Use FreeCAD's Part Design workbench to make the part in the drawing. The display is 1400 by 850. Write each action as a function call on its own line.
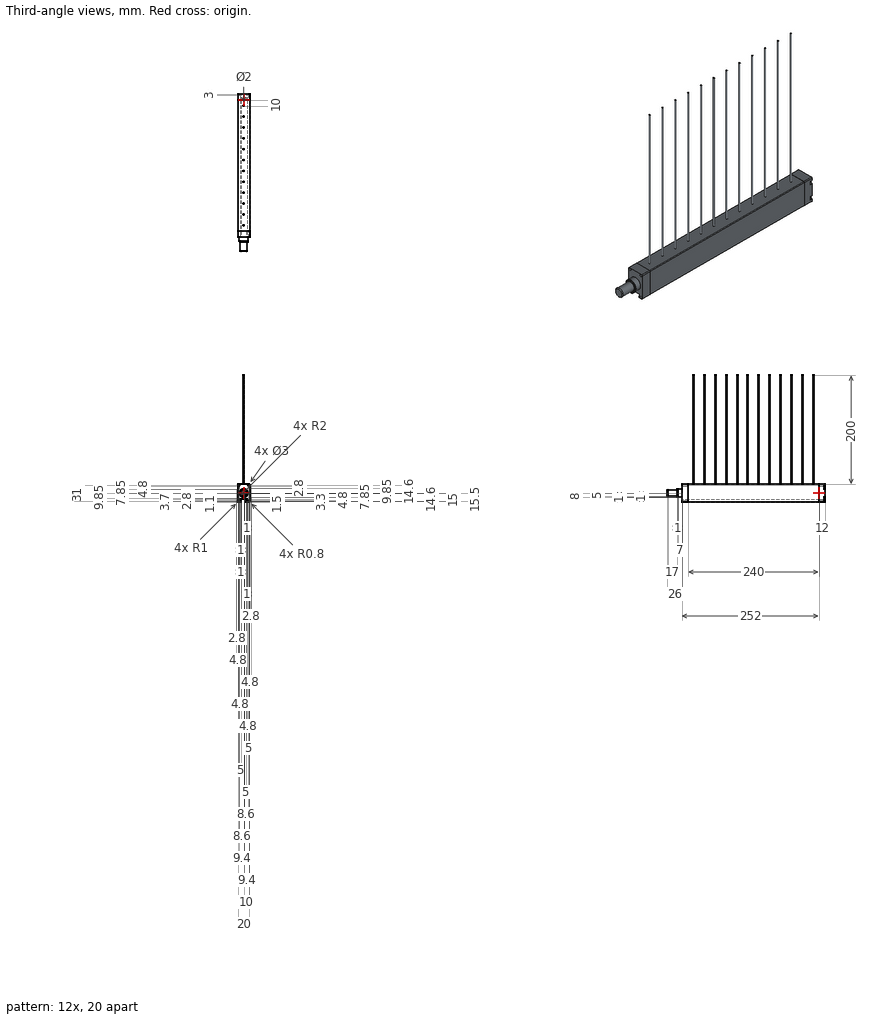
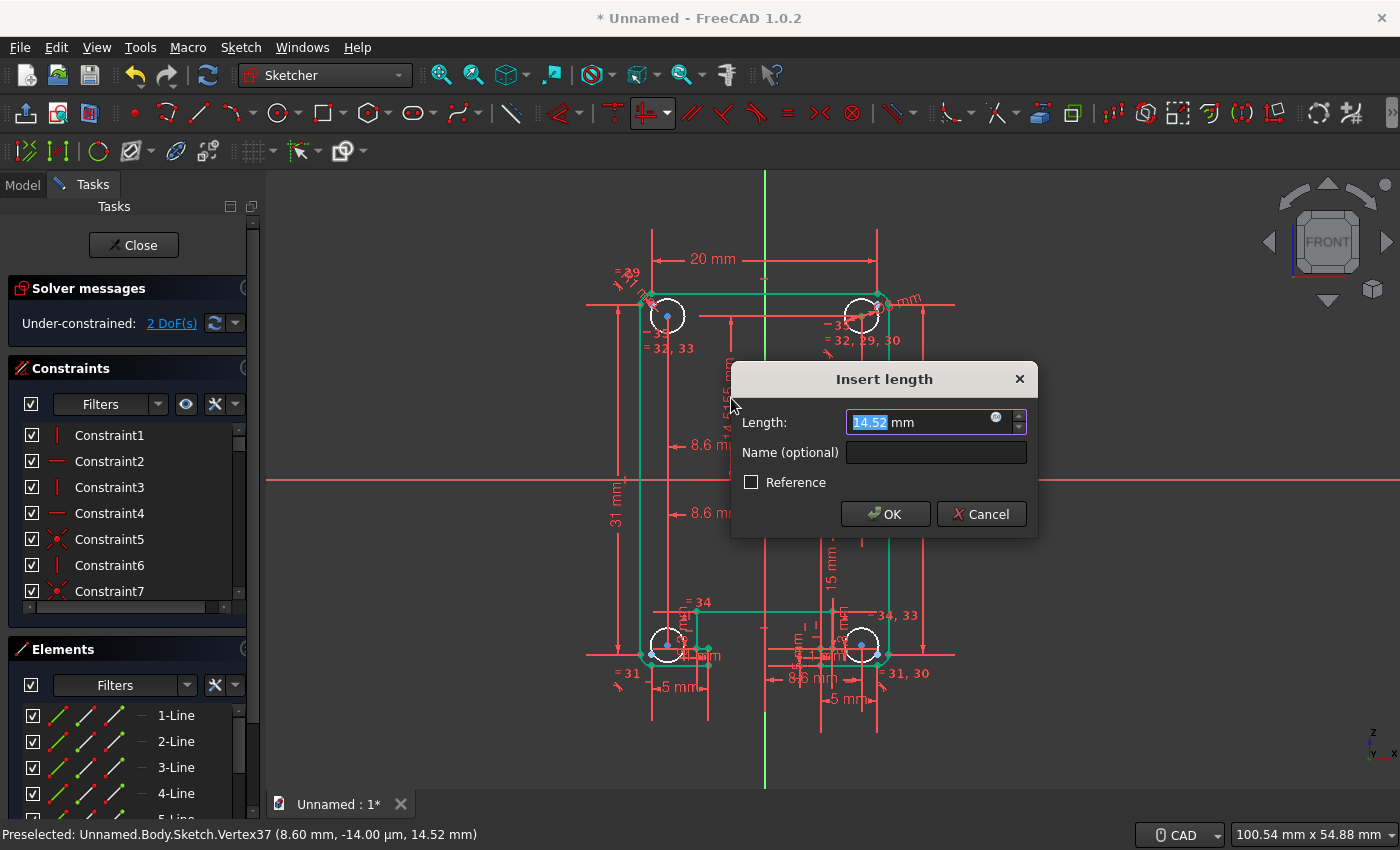
text(14.6)
key(Return)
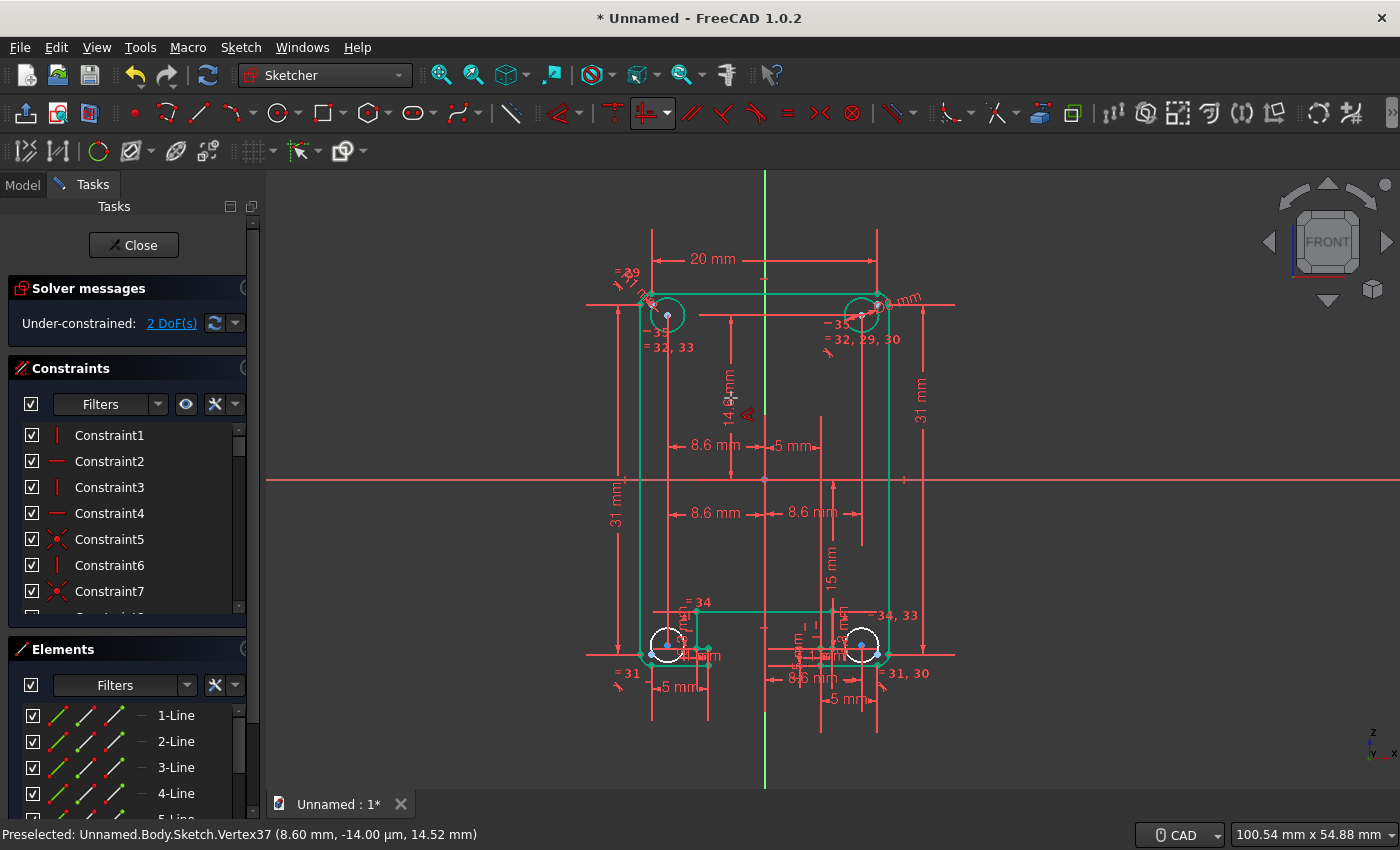
click(862, 645)
click(731, 562)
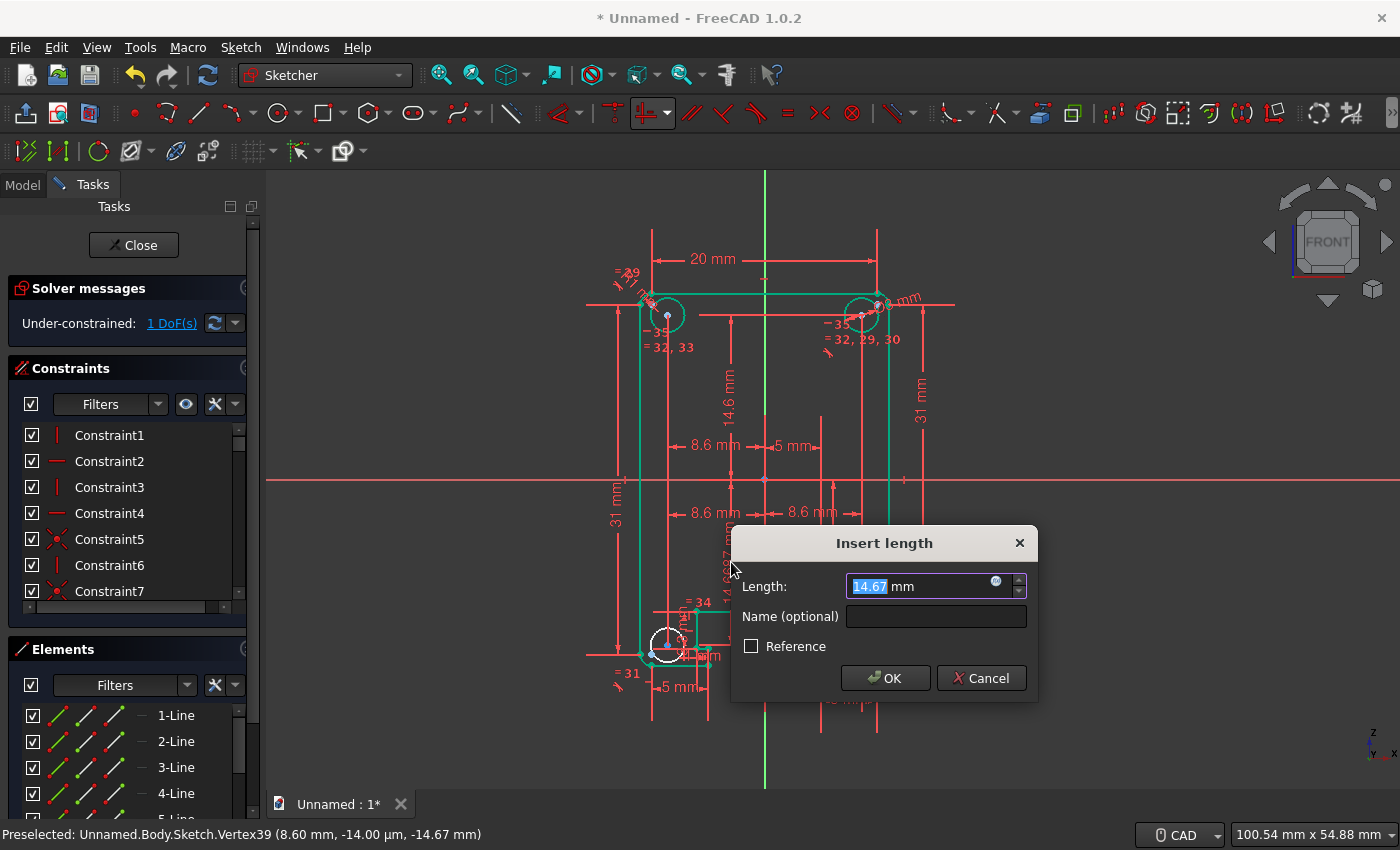
text(14.6)
key(Return)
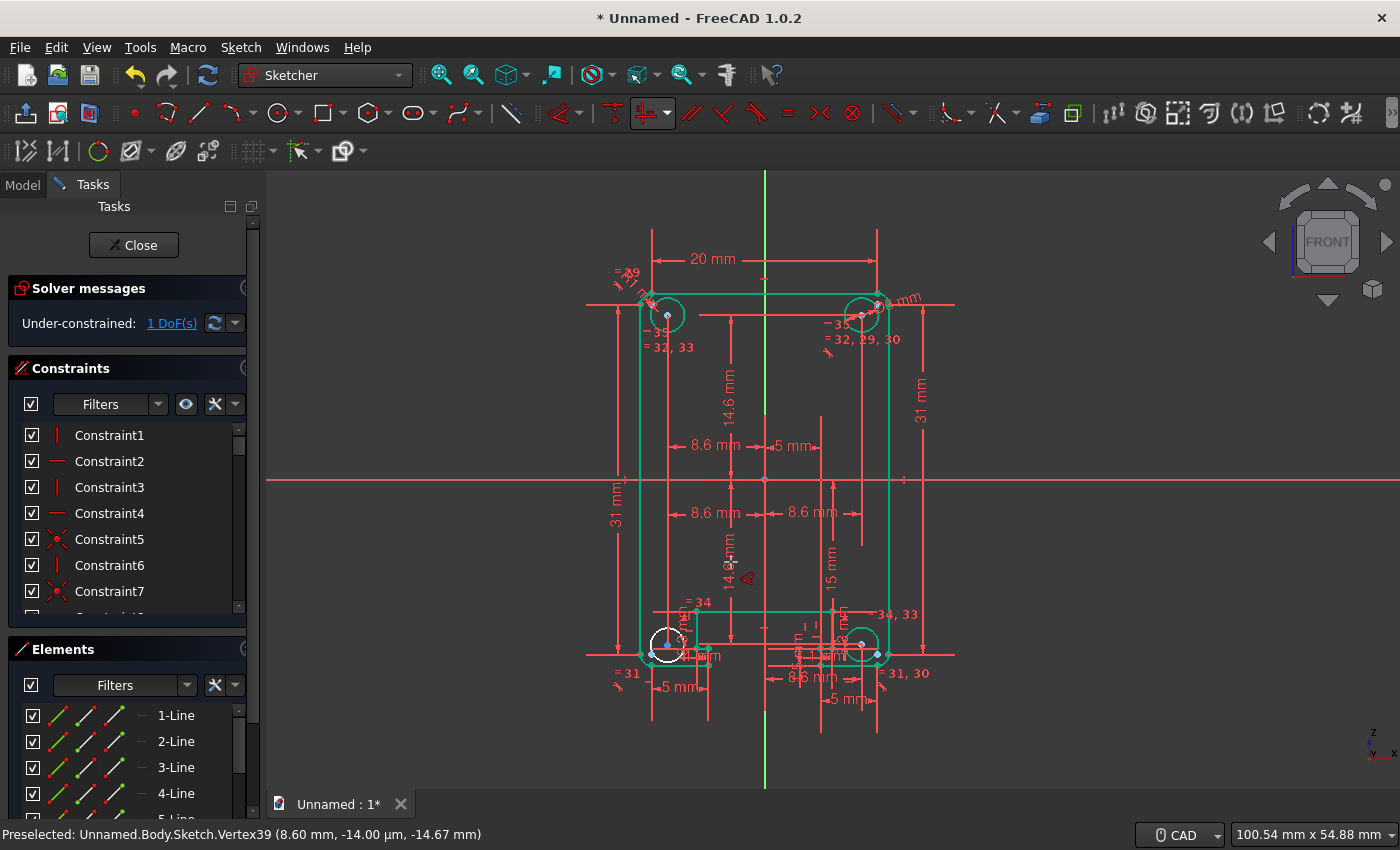
click(668, 645)
click(610, 562)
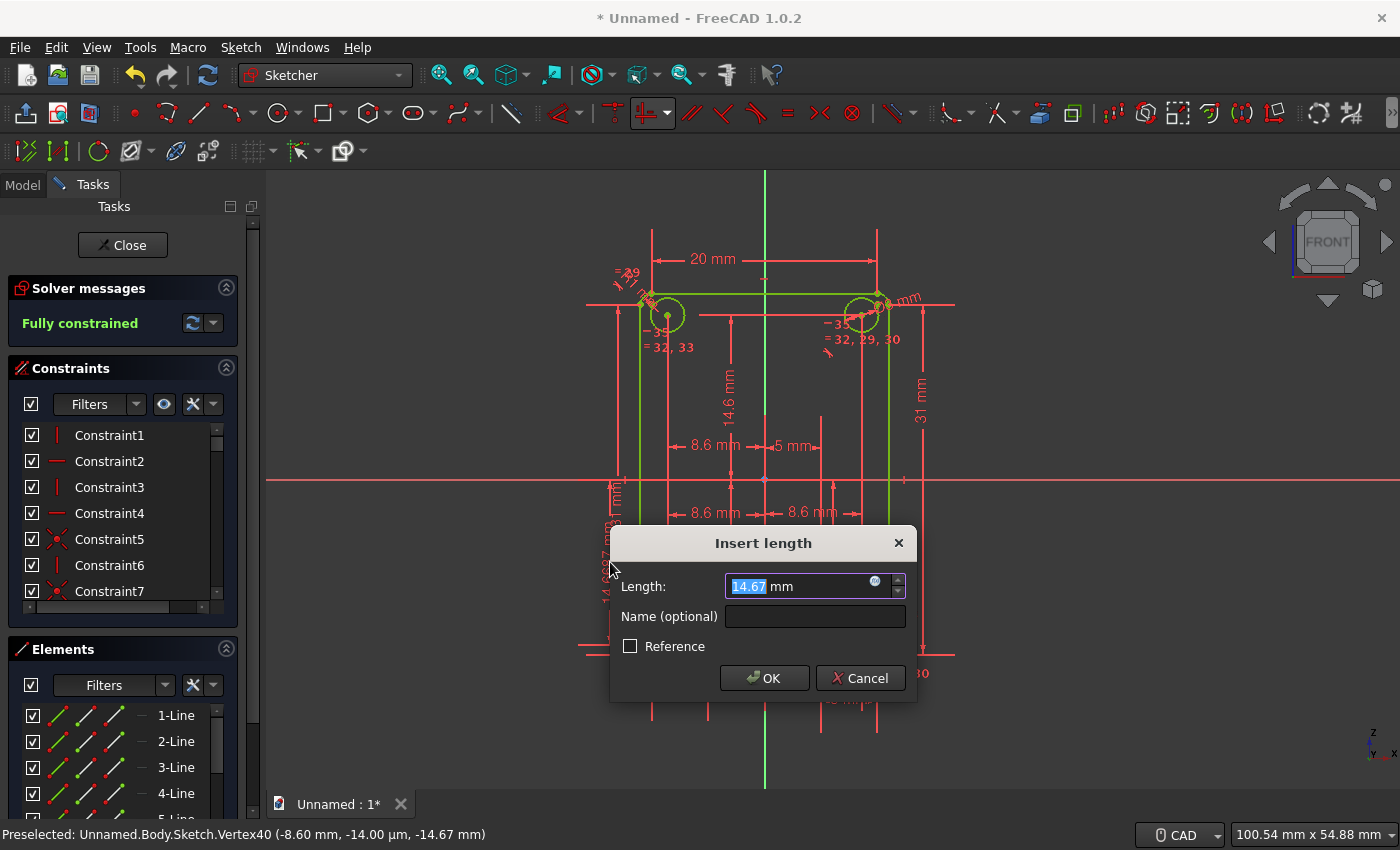
text(14.6)
key(Return)
key(Escape)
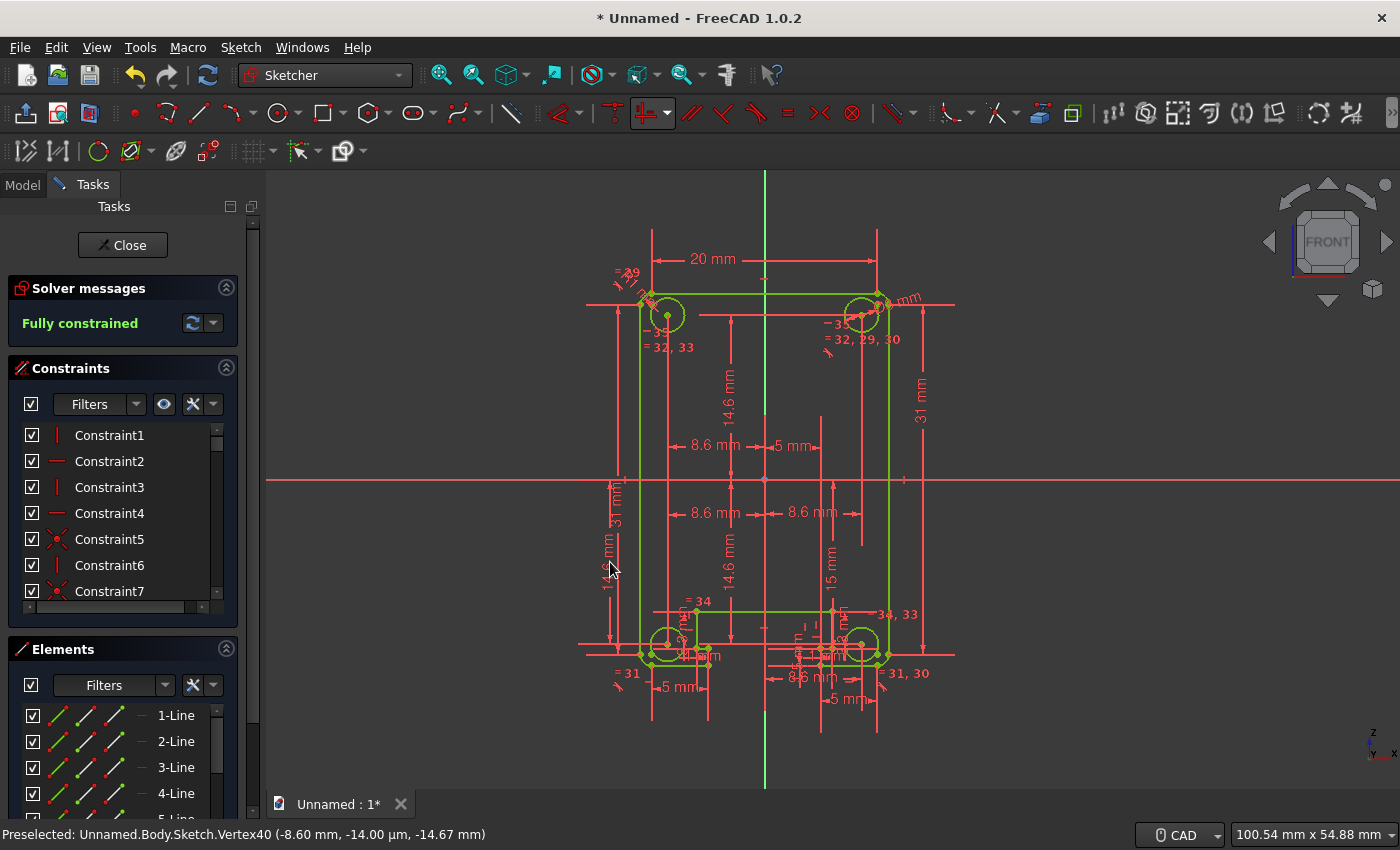
click(123, 245)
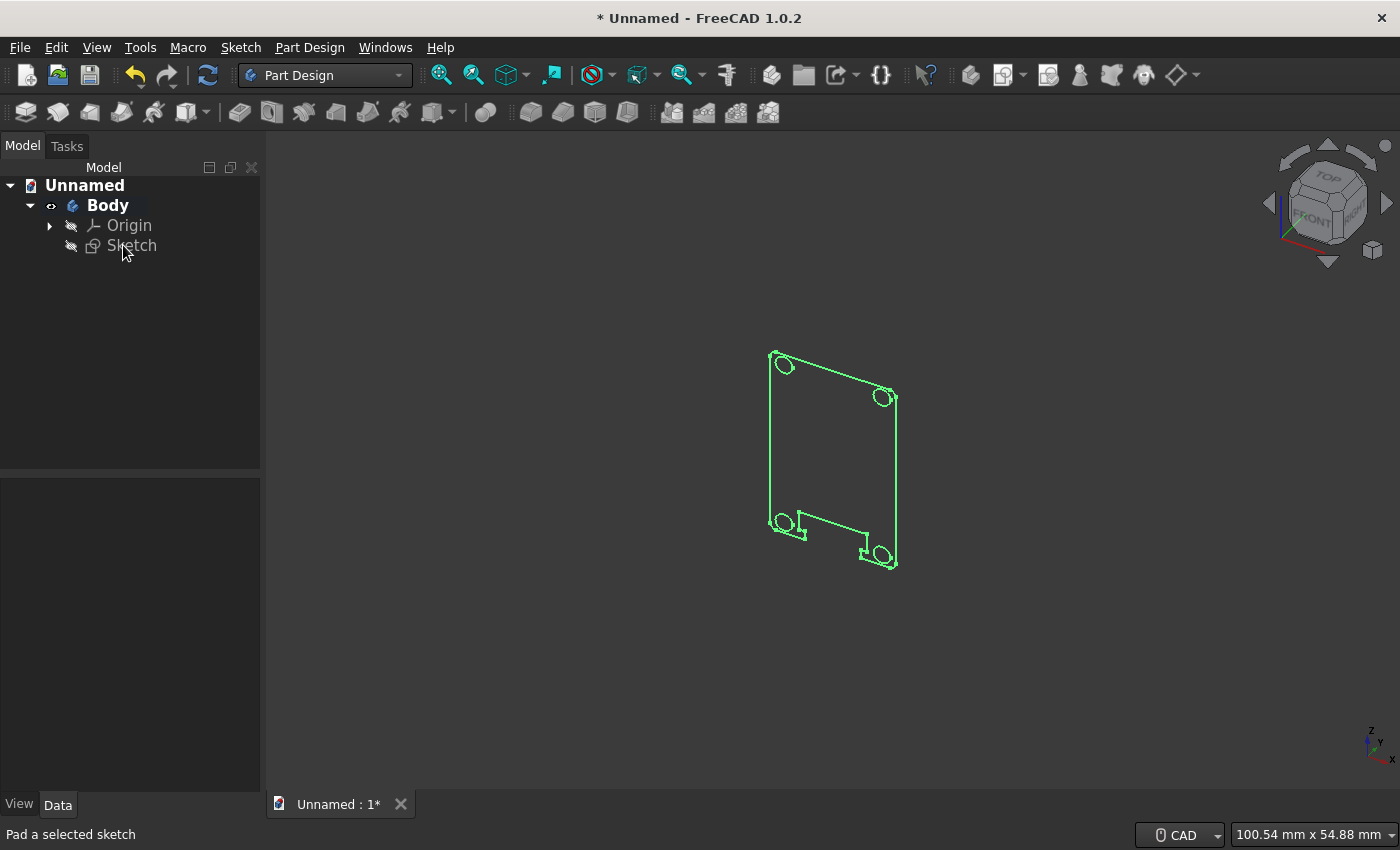
click(26, 112)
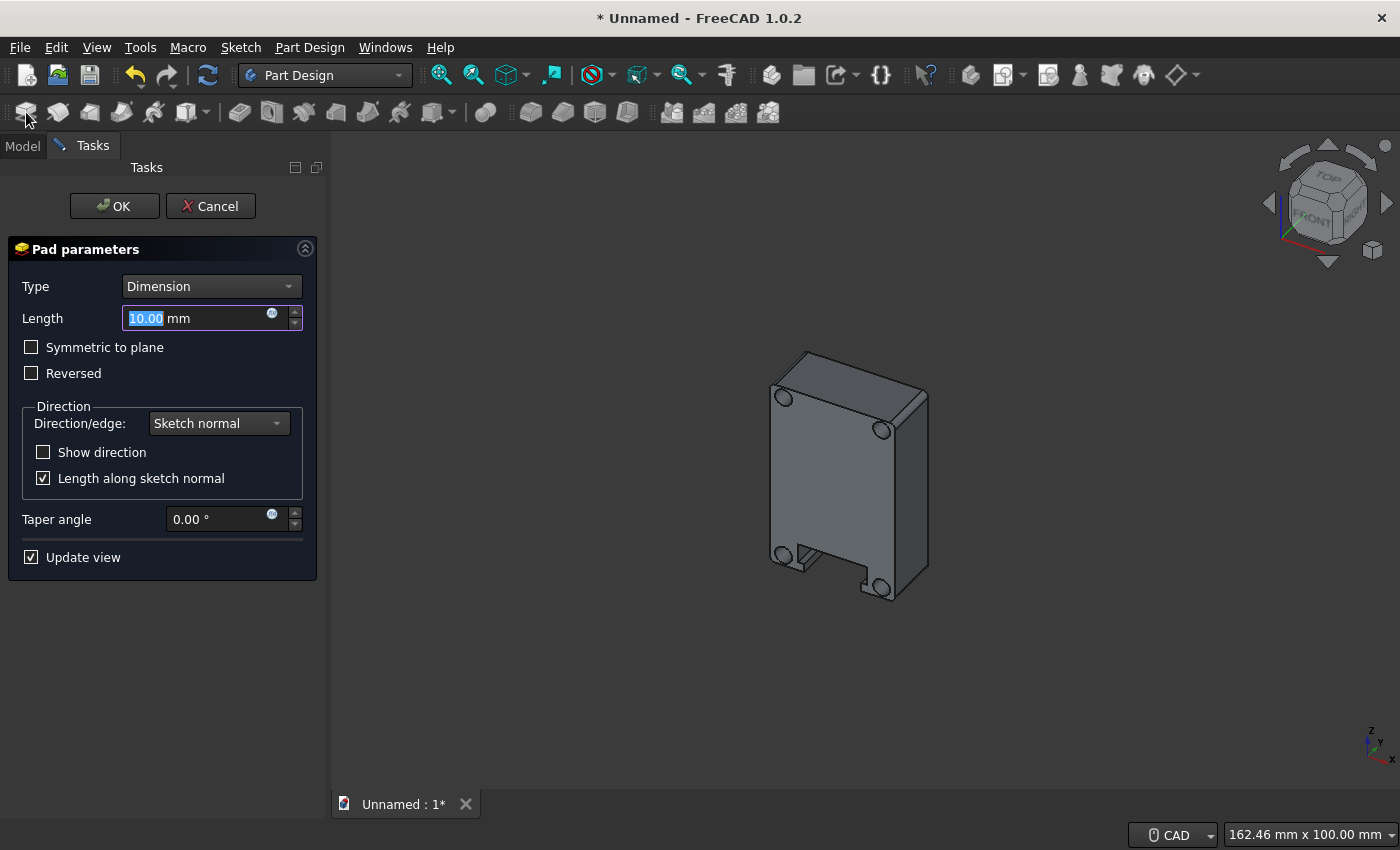
text(12)
key(Tab)